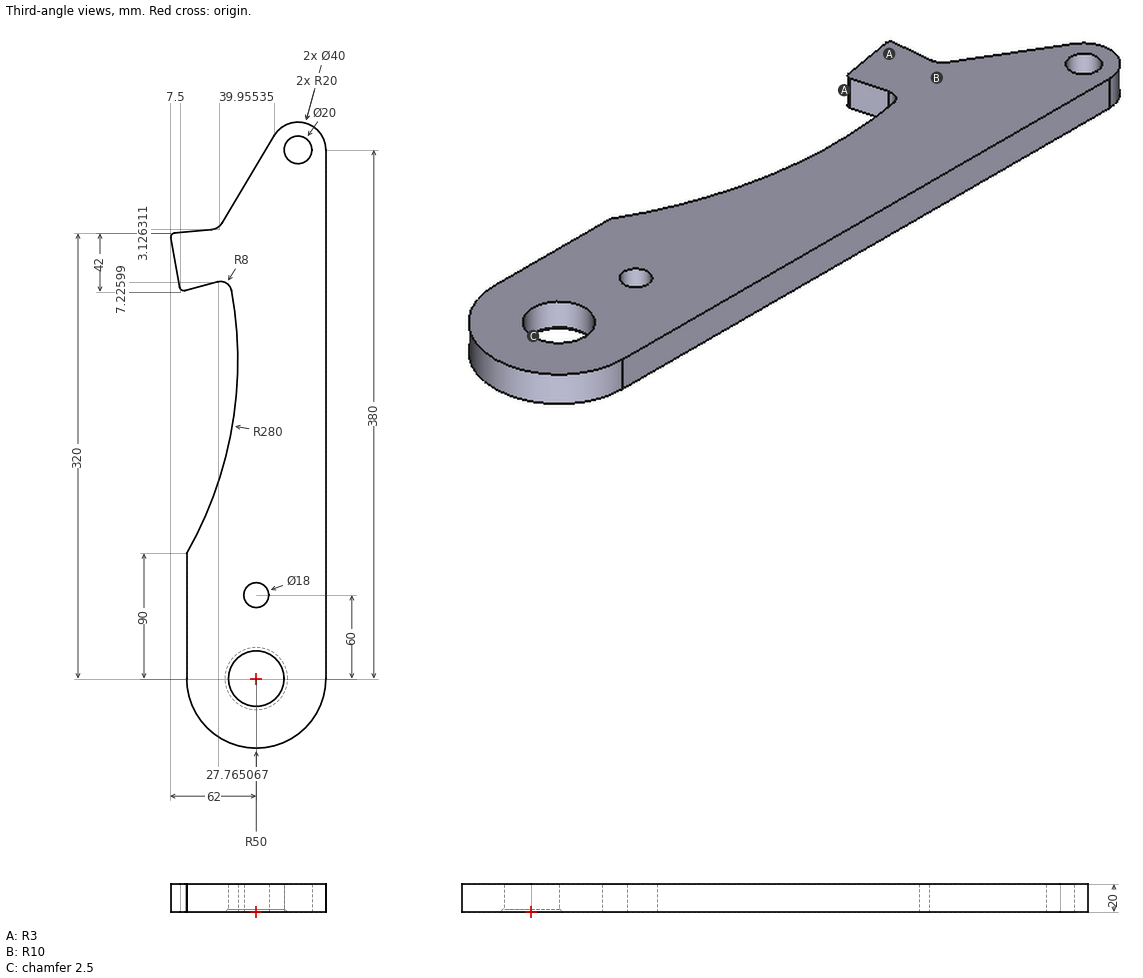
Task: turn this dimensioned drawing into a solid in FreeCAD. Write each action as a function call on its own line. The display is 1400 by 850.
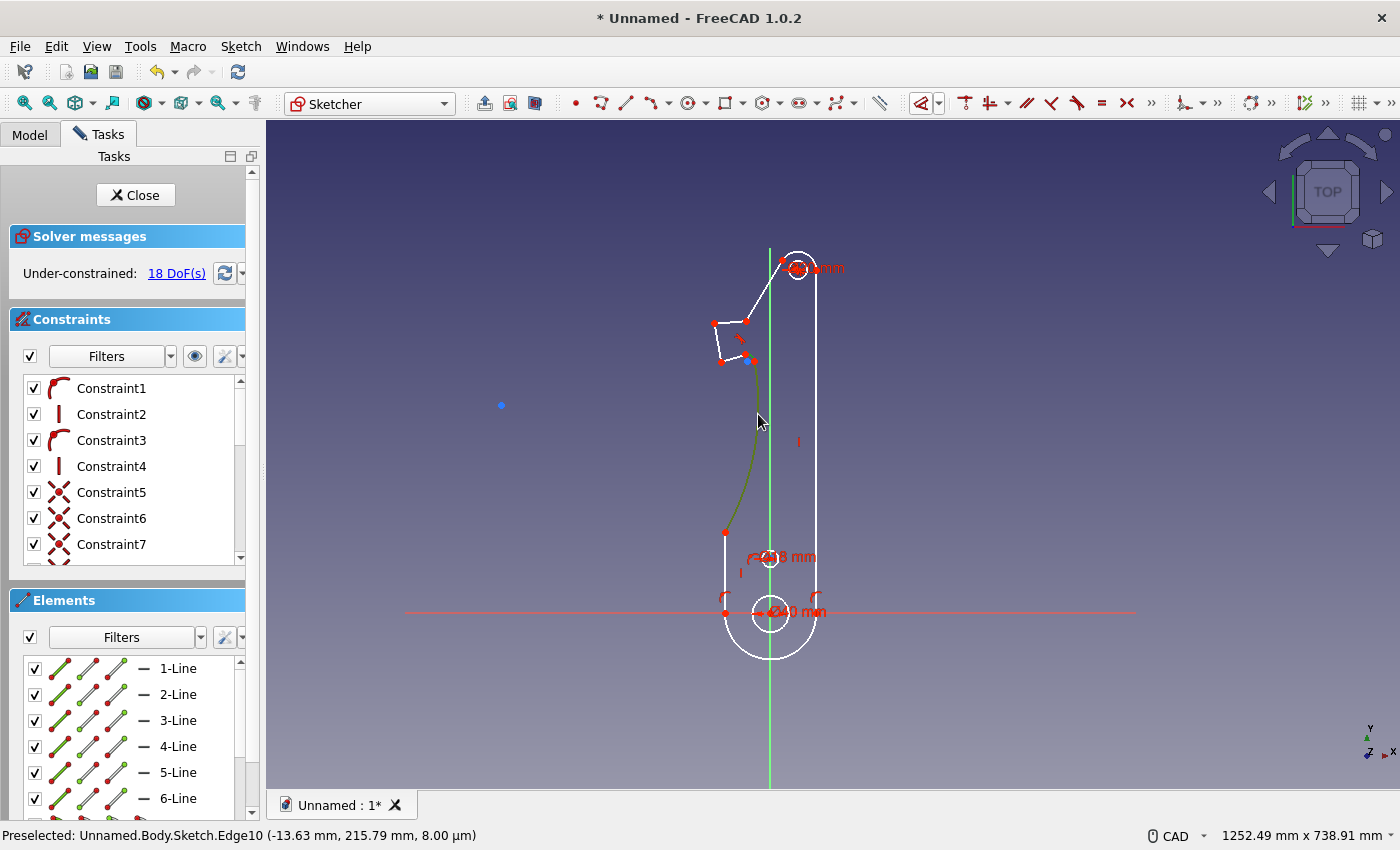
click(1077, 104)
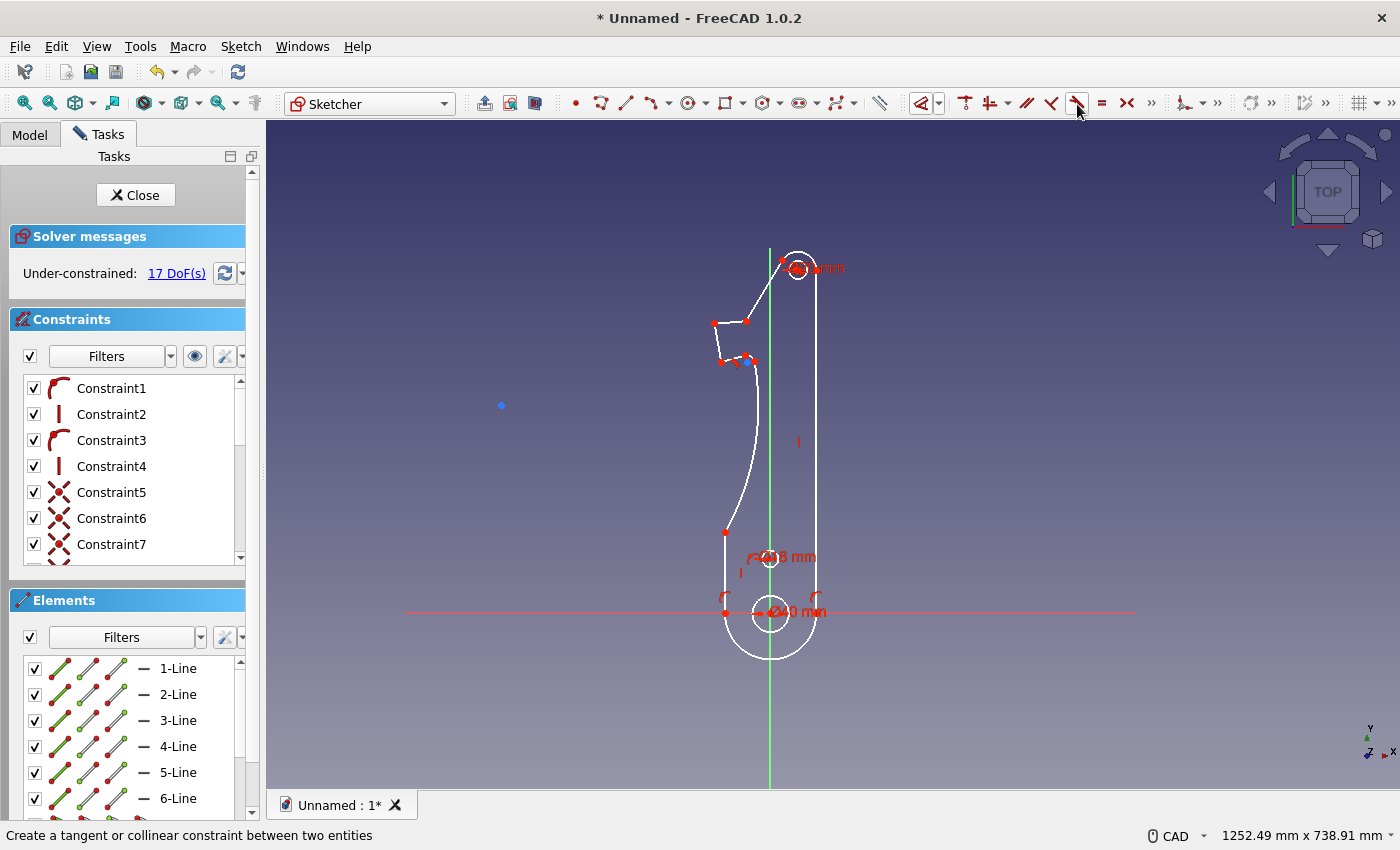
scroll(770, 613, up, 9)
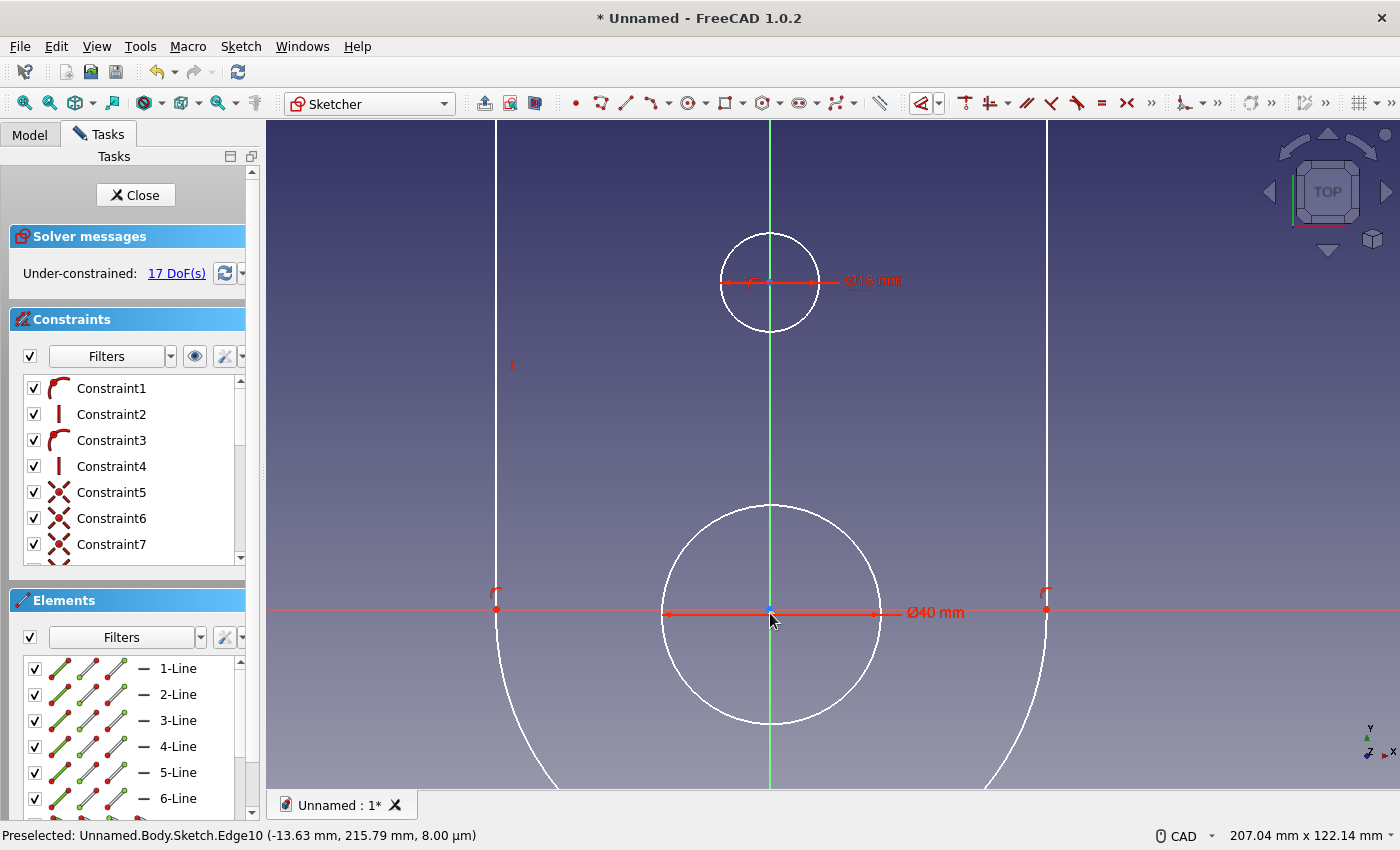
drag(760, 600, 781, 625)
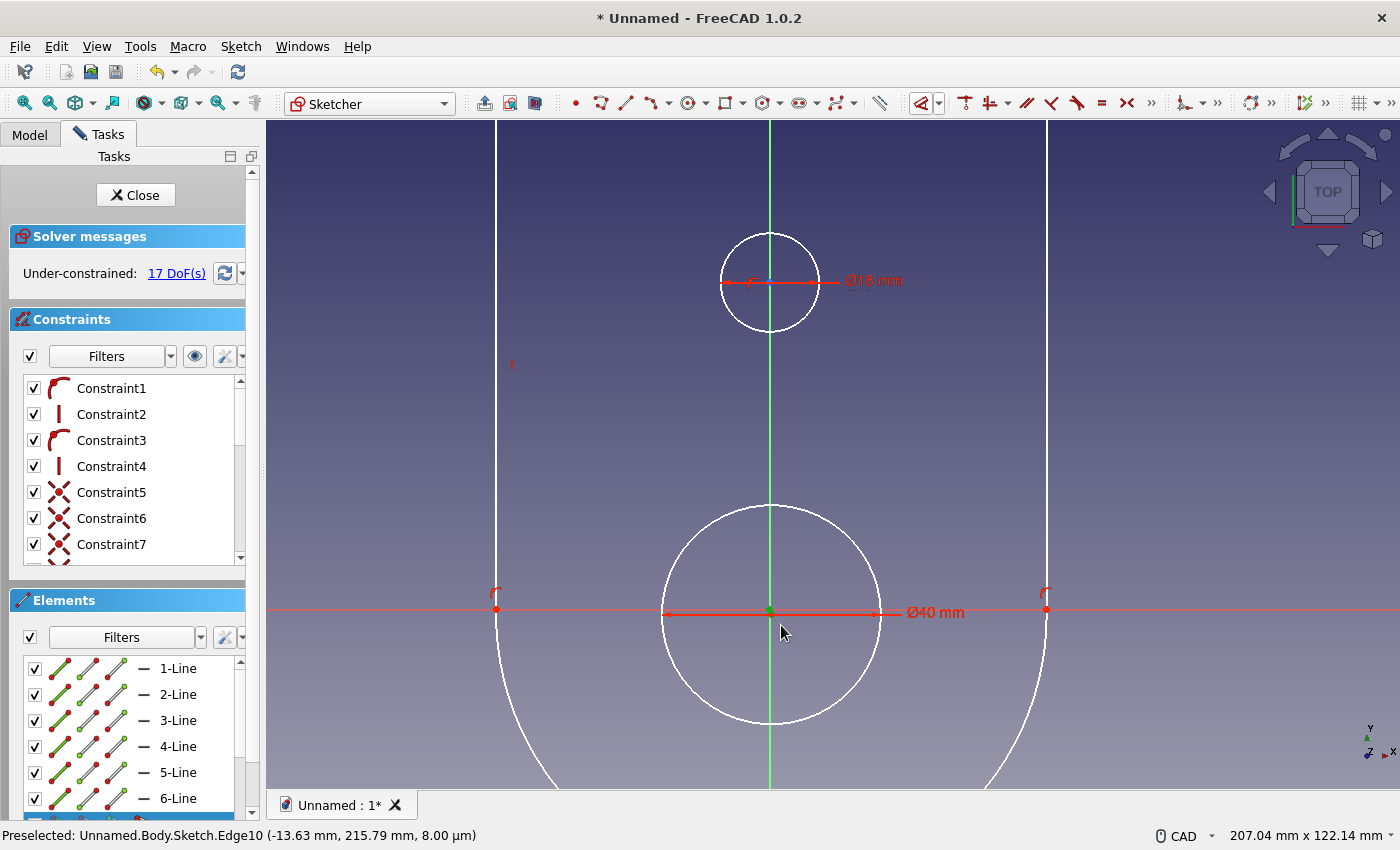
key(c)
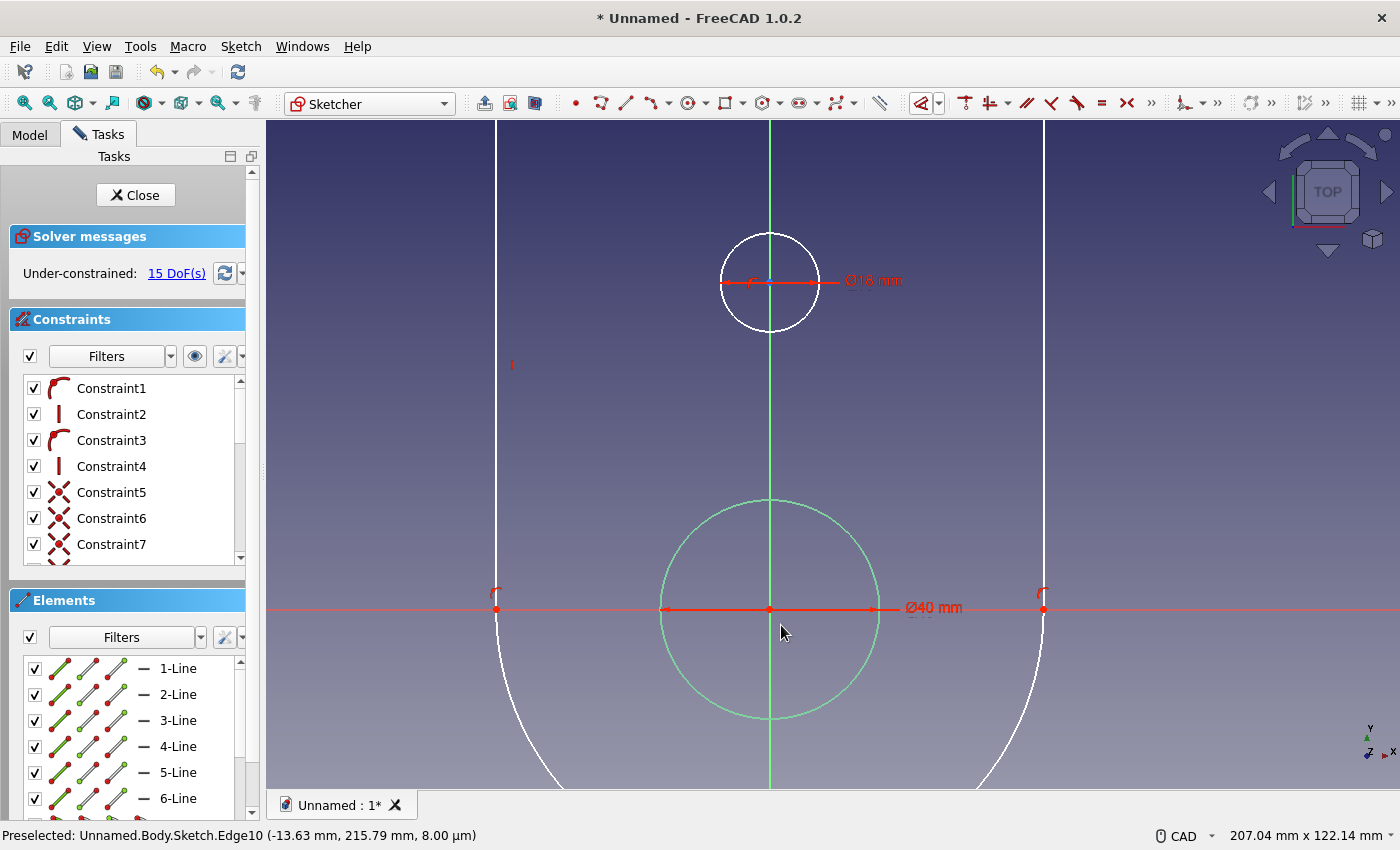
click(920, 104)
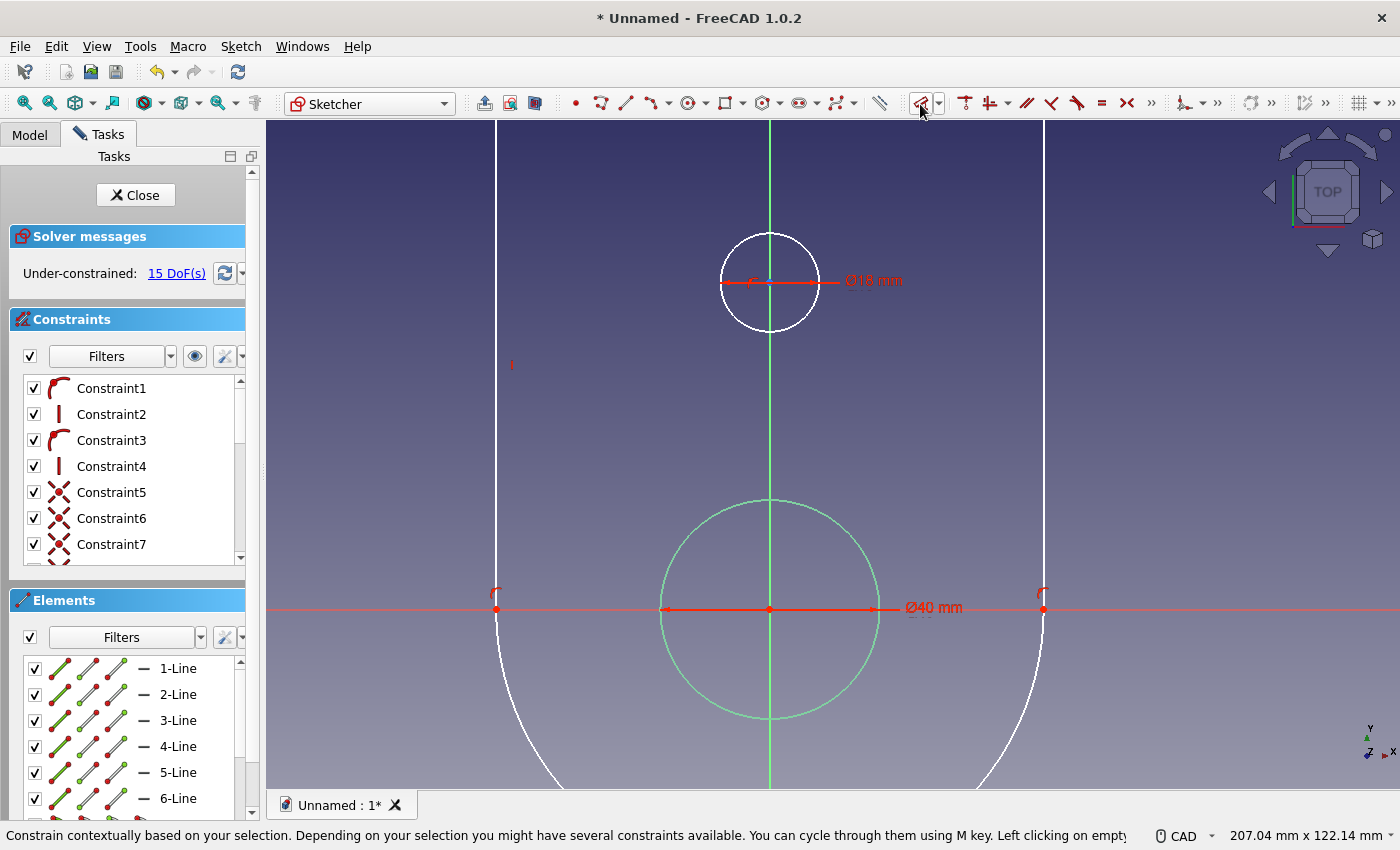
scroll(770, 613, down, 9)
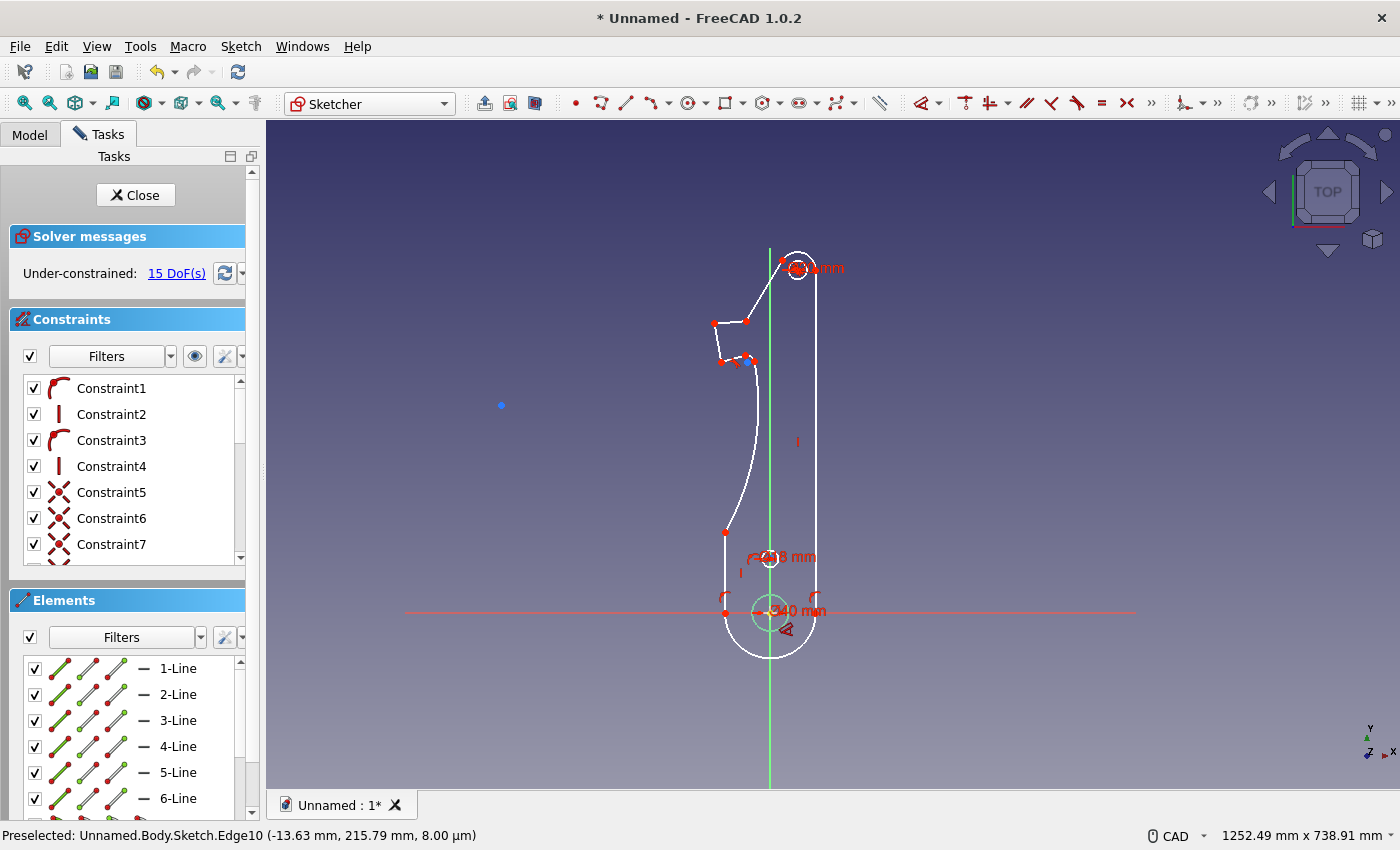
click(744, 650)
click(725, 676)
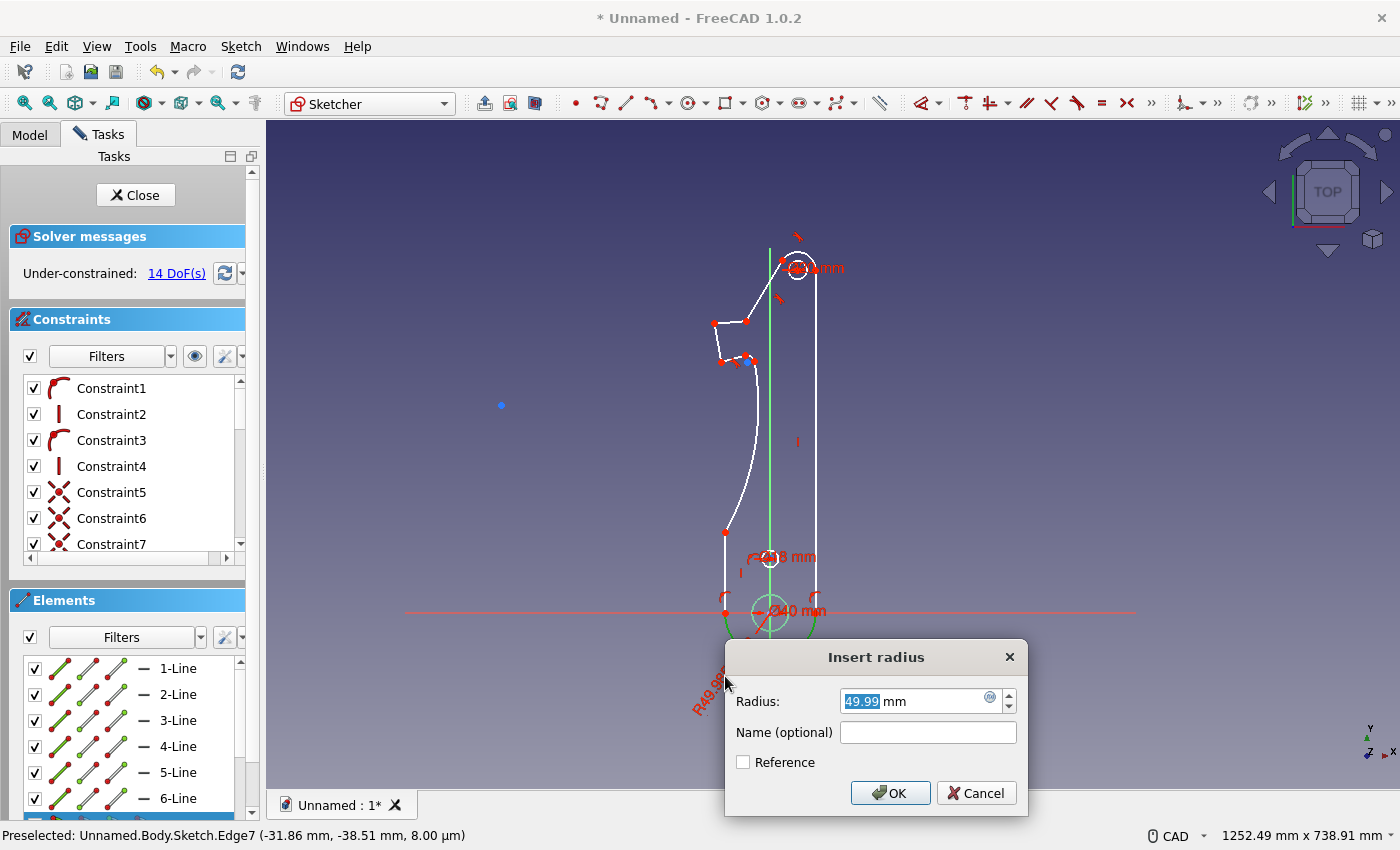
text(50)
key(Return)